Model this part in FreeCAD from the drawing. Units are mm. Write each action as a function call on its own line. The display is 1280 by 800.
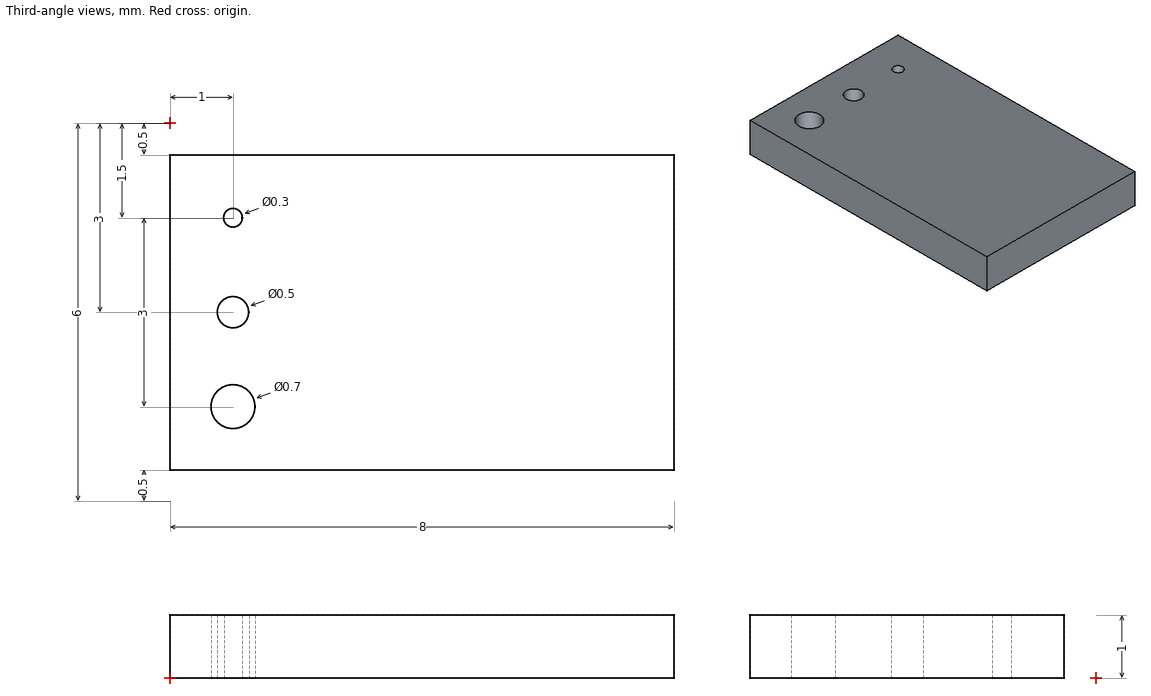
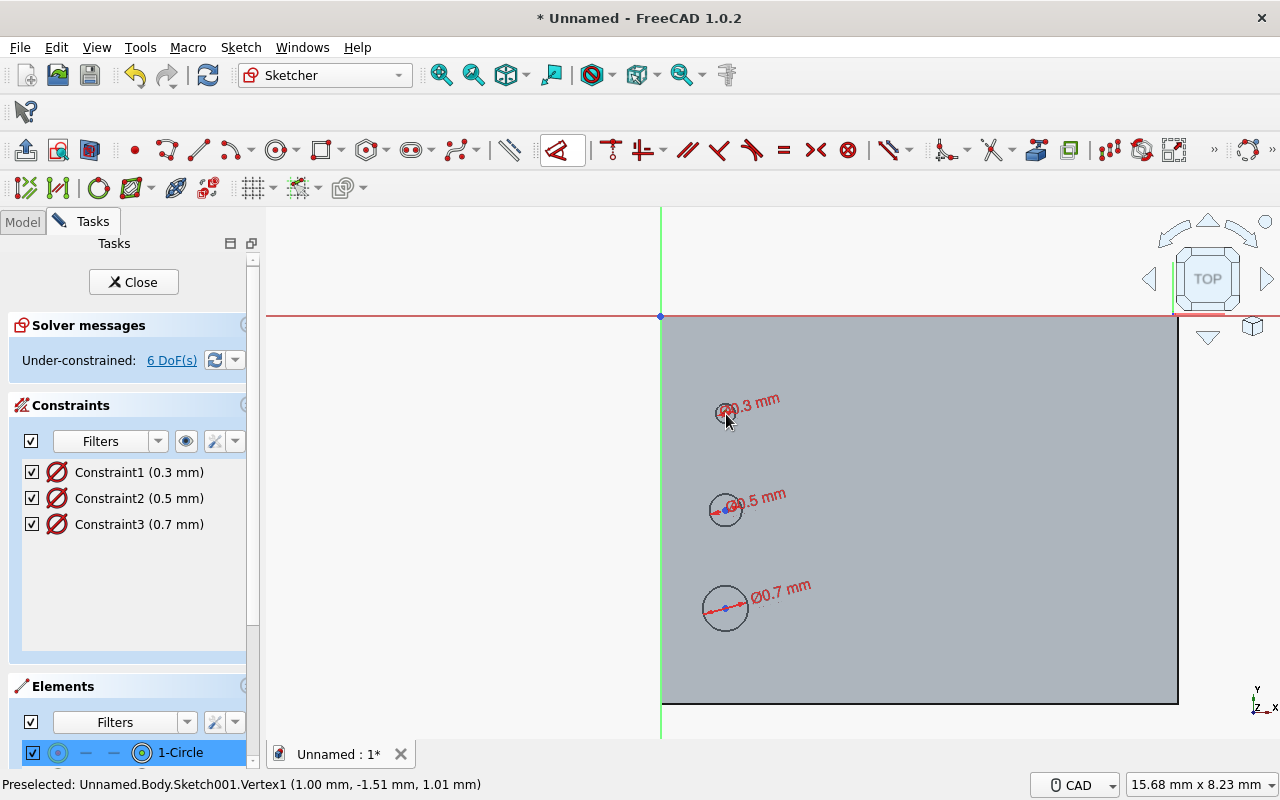
click(580, 150)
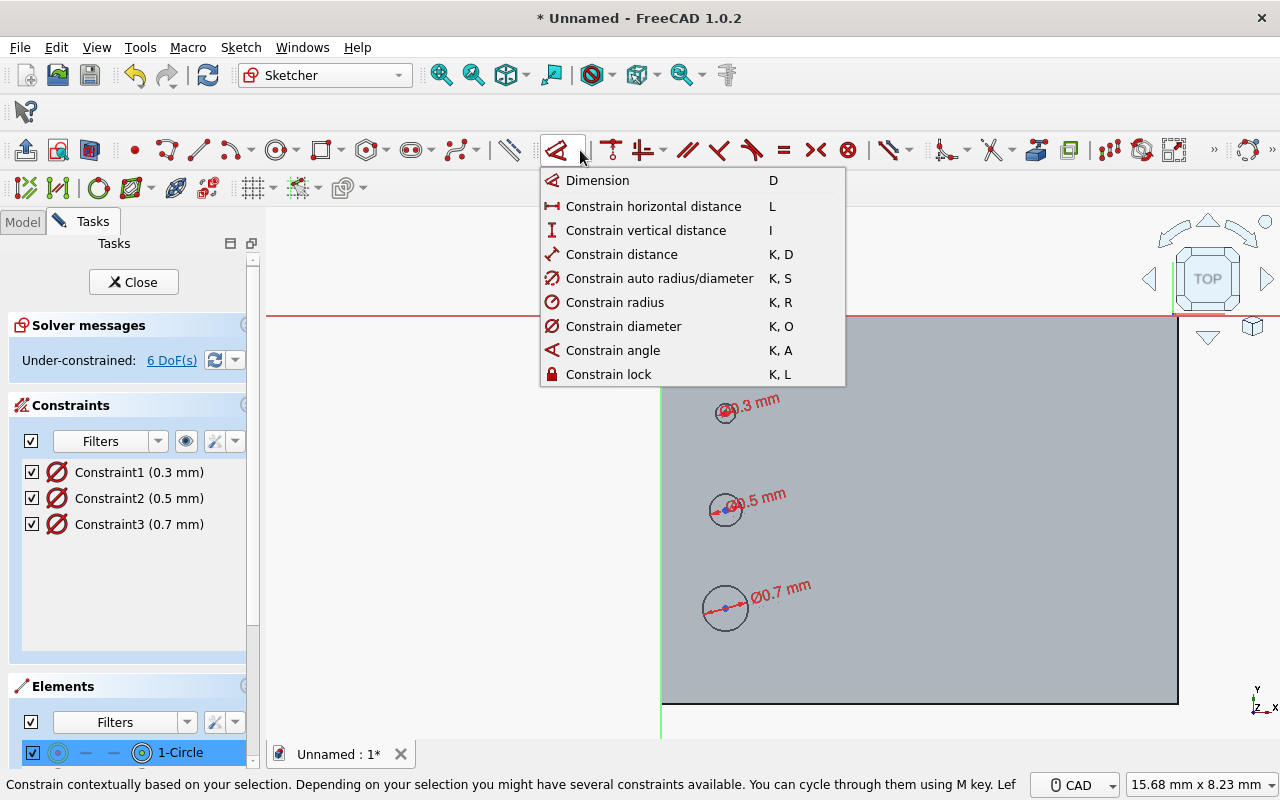
click(693, 206)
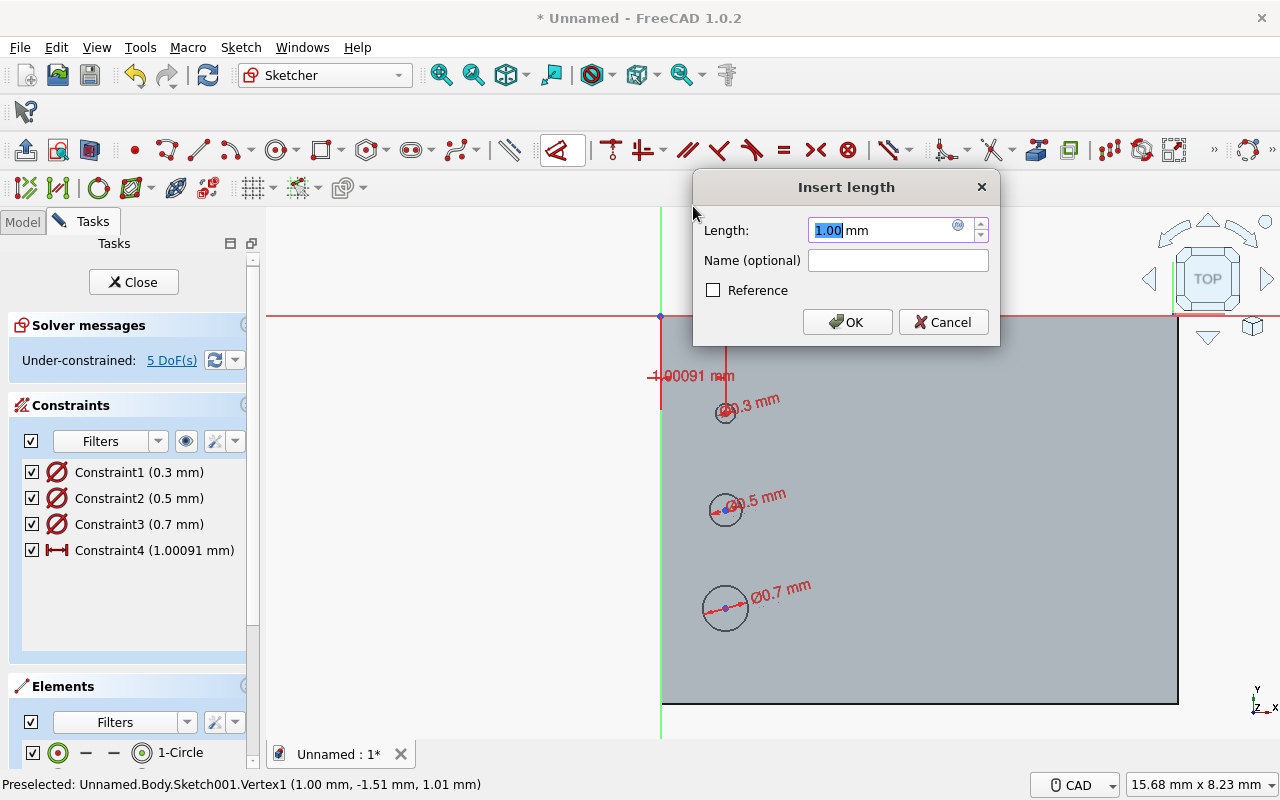
text(1)
key(Return)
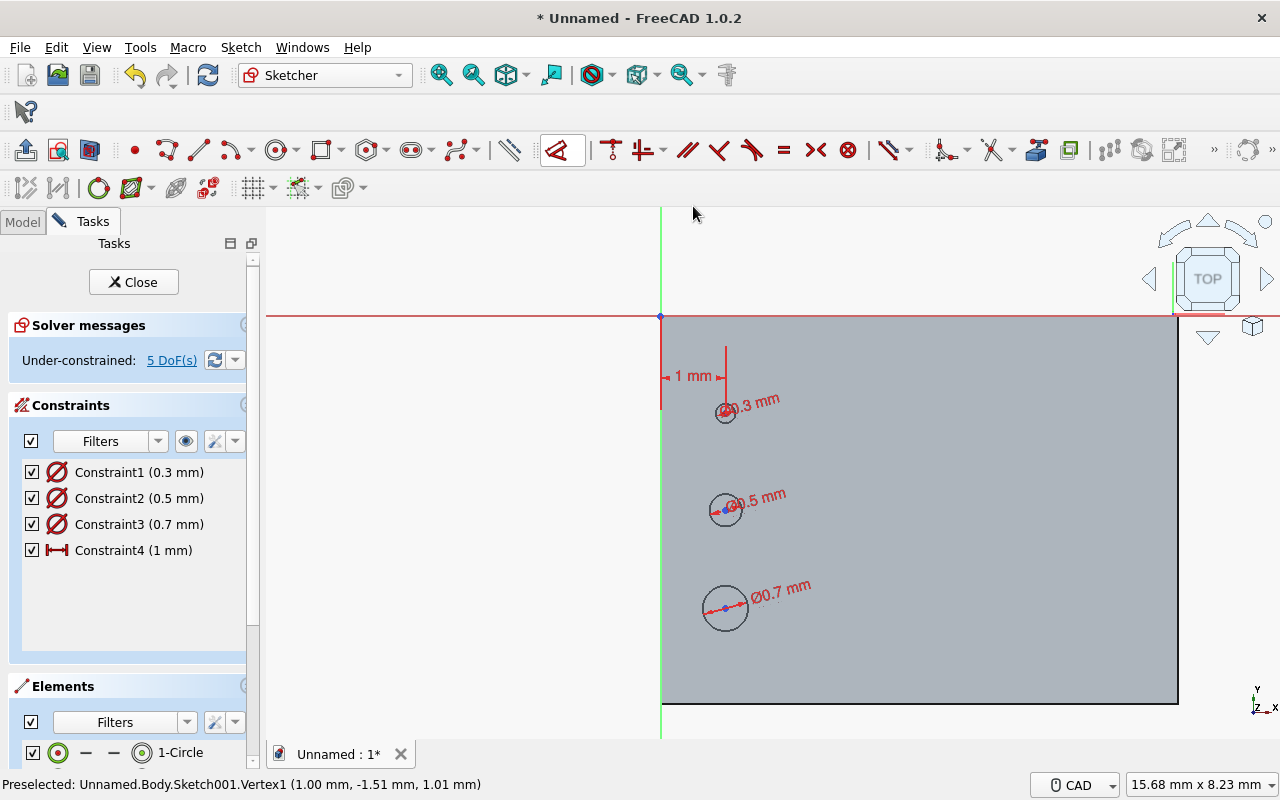
click(726, 510)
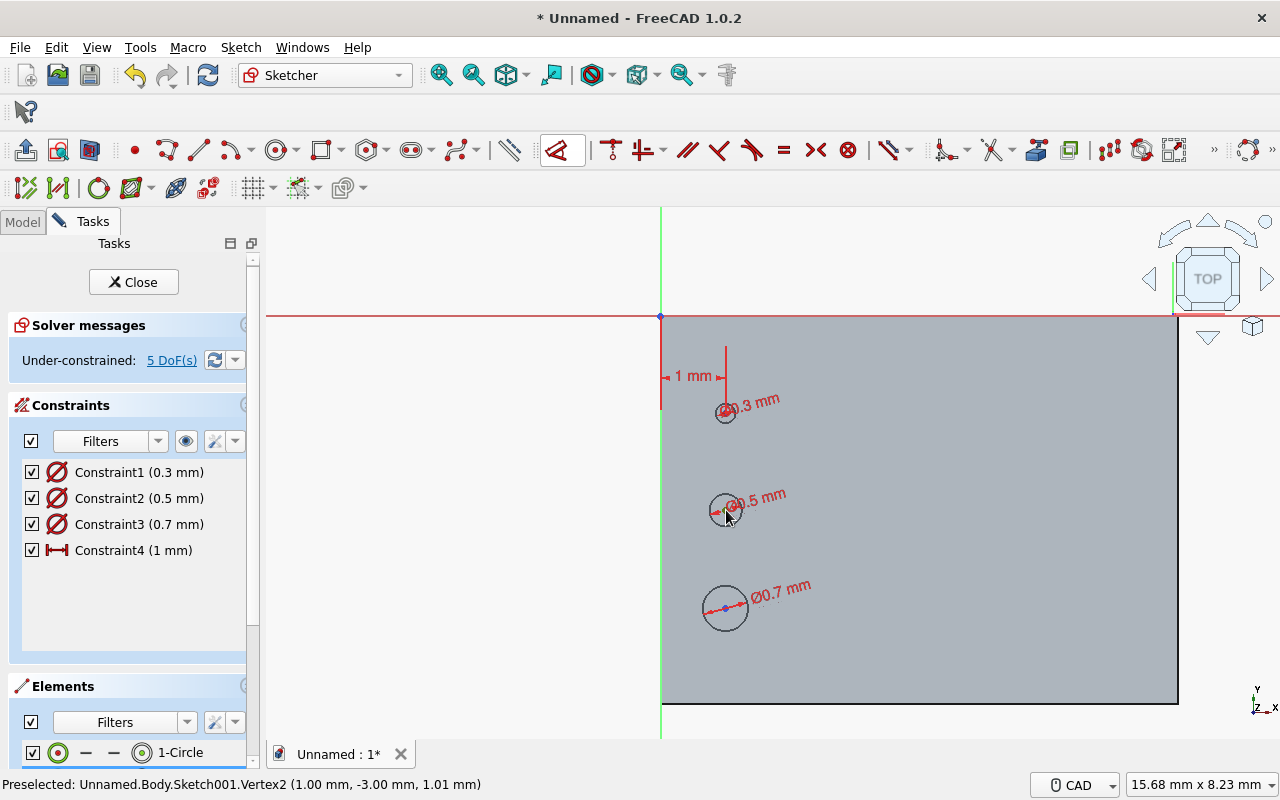
key(l)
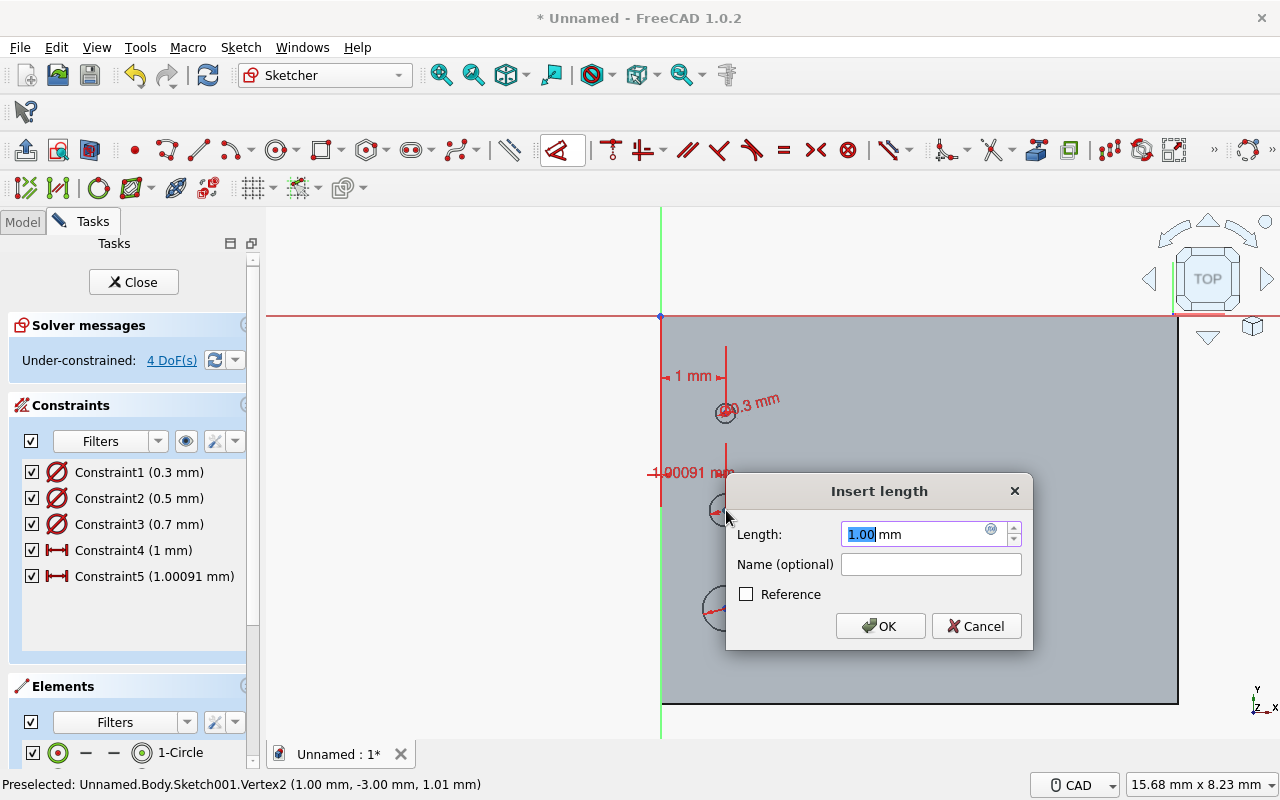
text(1)
key(Return)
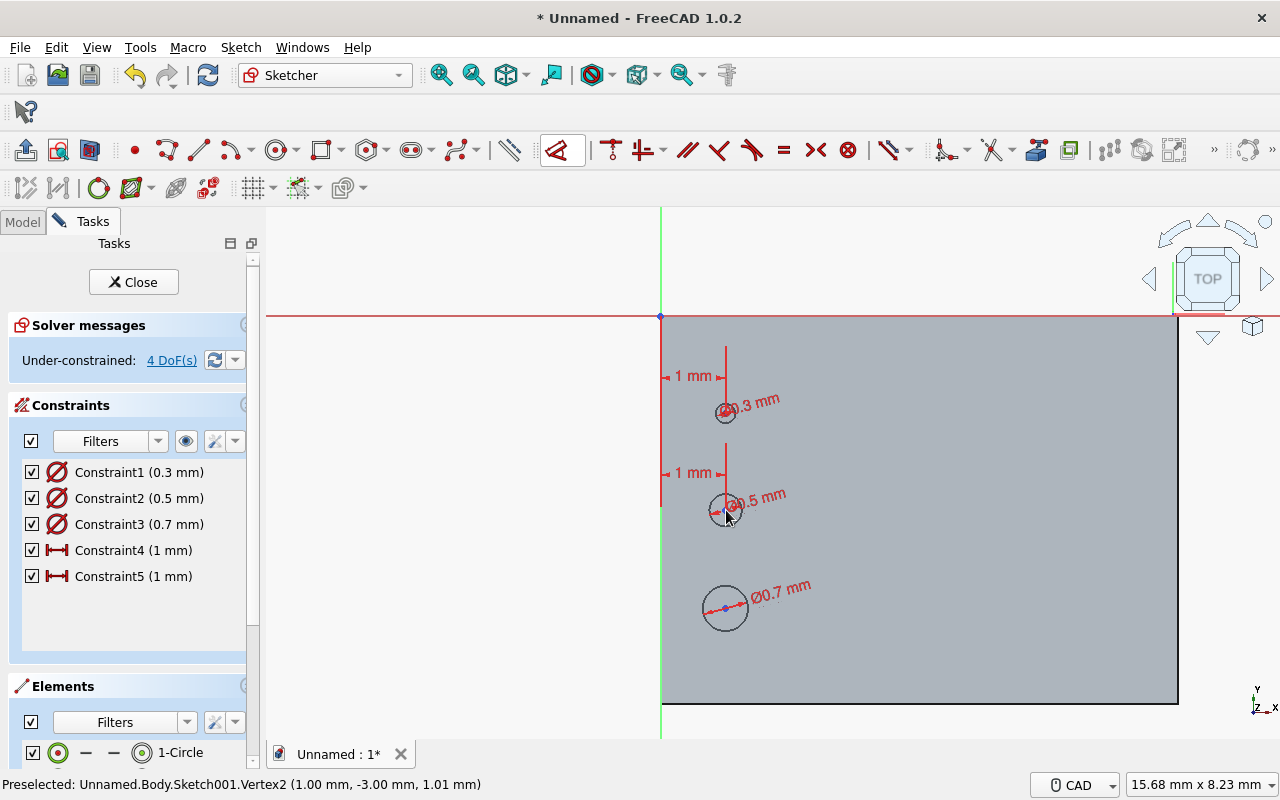
click(726, 510)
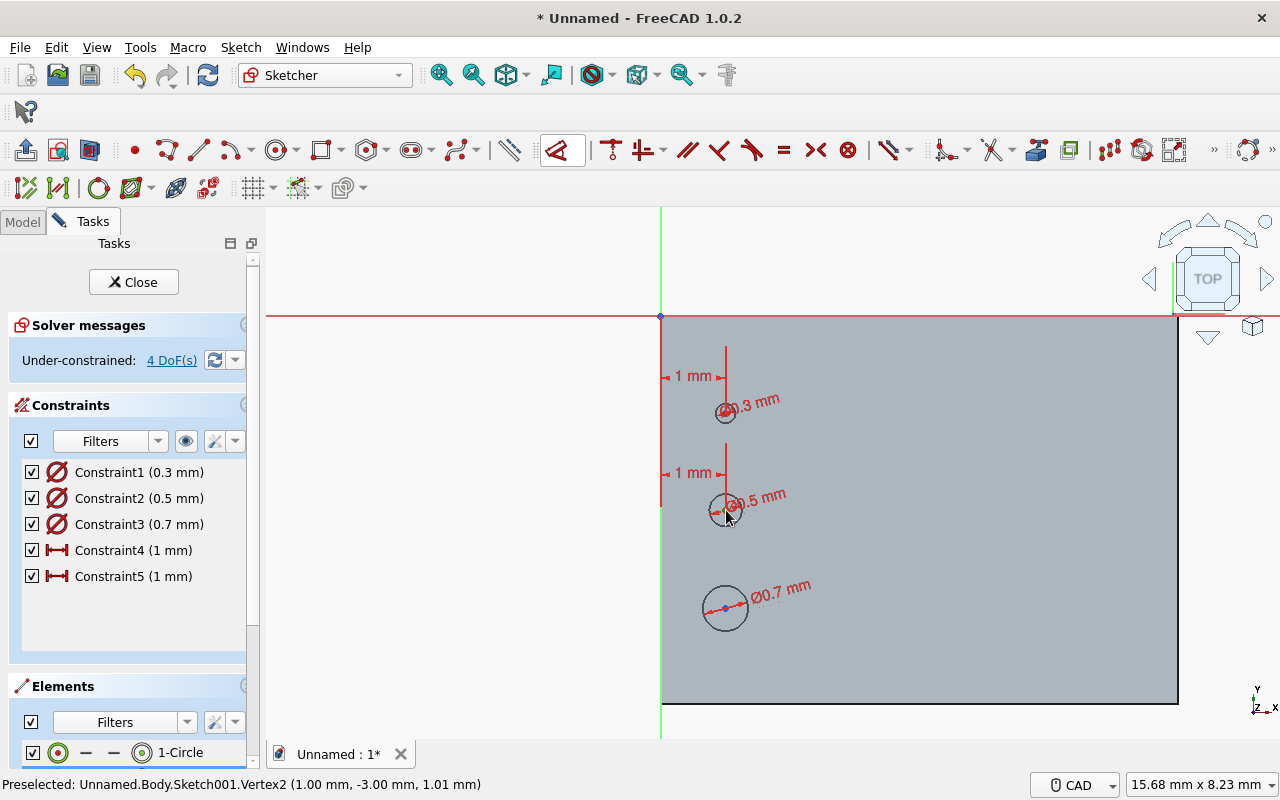
key(i)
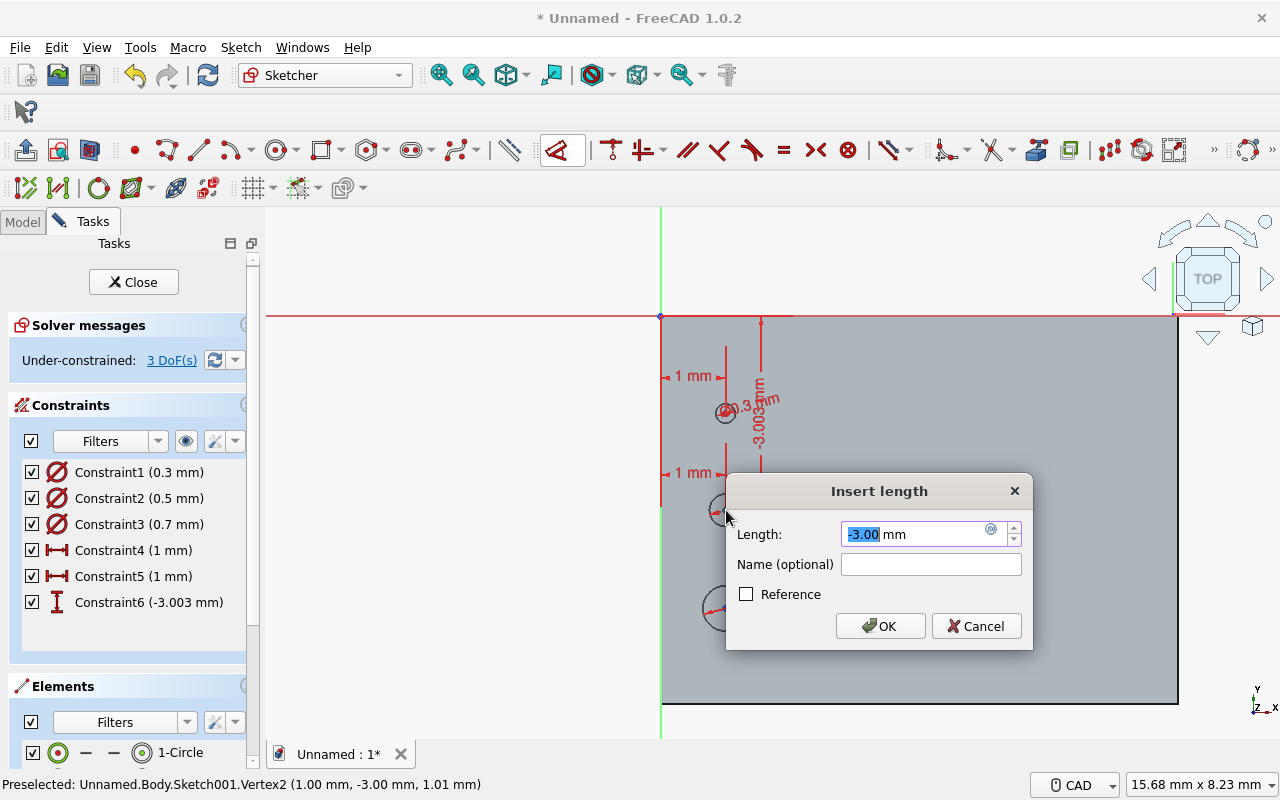
text(-3)
key(Return)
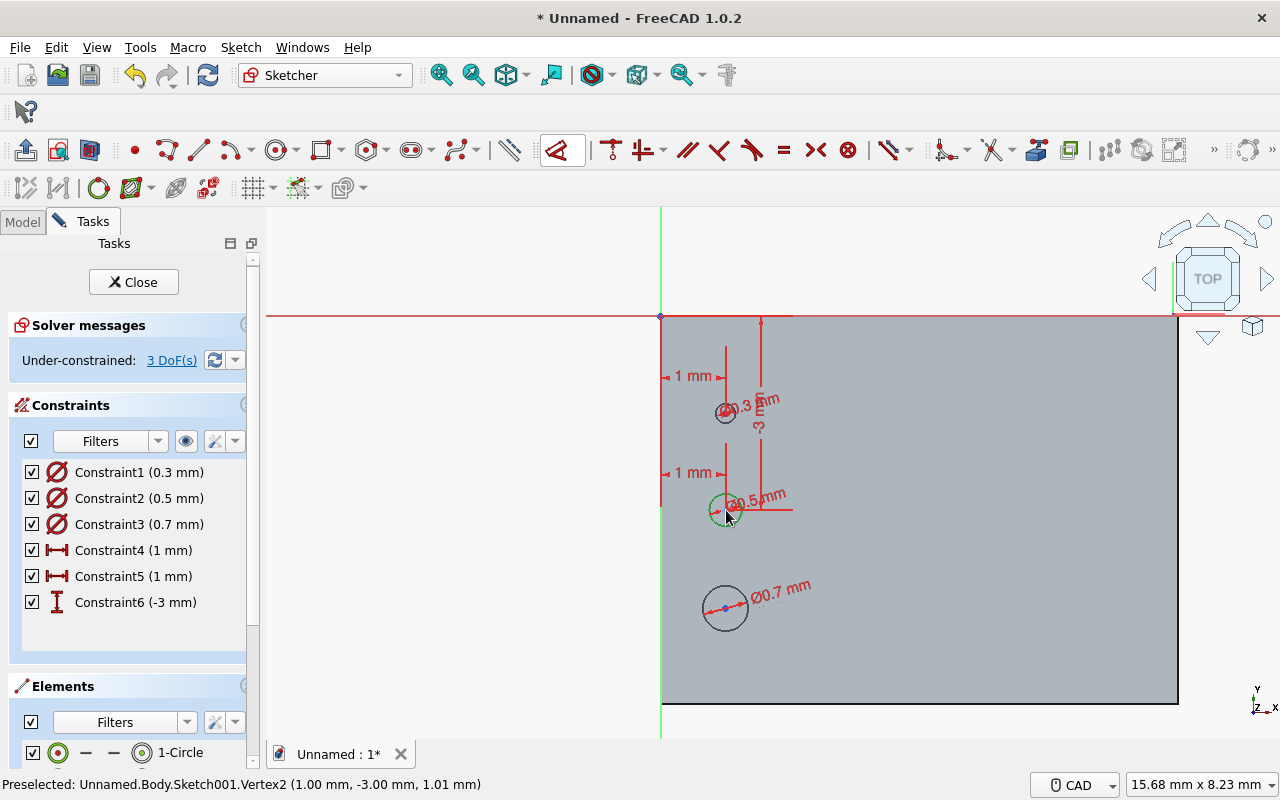
click(725, 608)